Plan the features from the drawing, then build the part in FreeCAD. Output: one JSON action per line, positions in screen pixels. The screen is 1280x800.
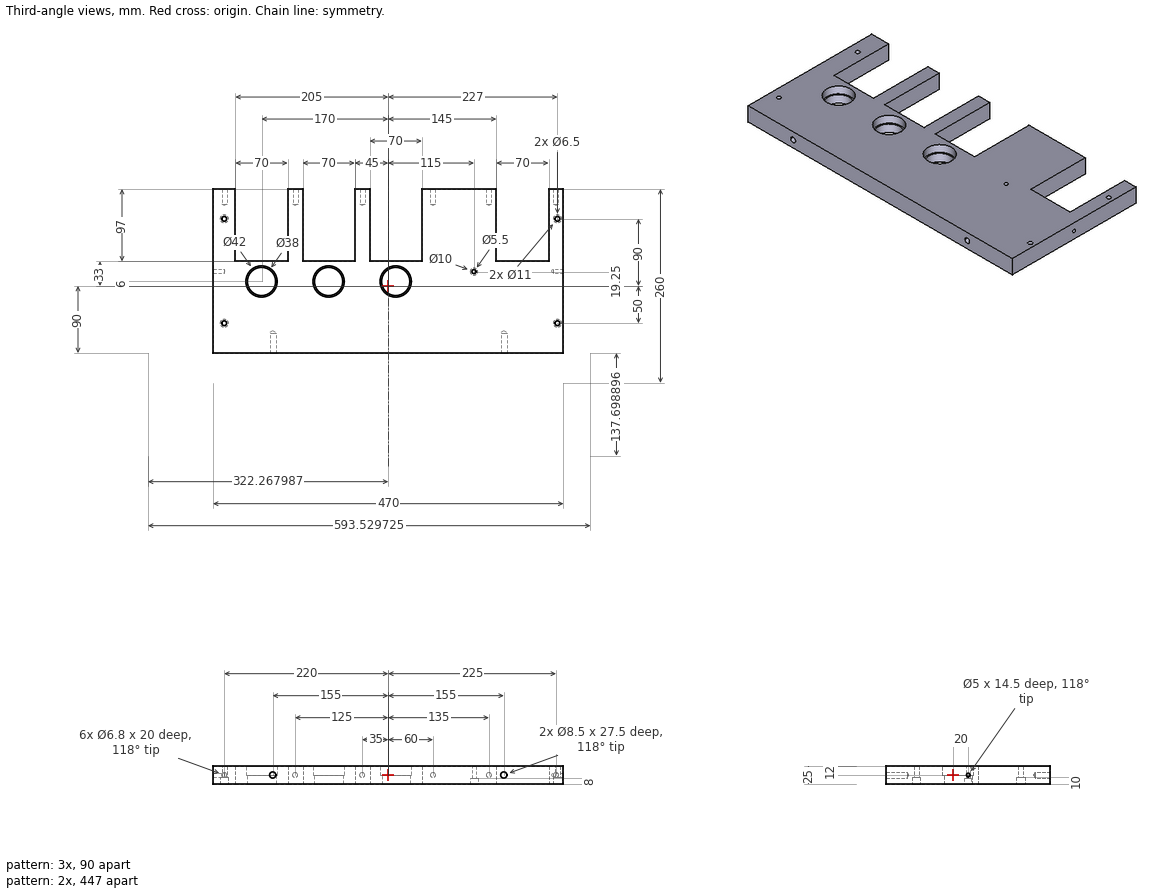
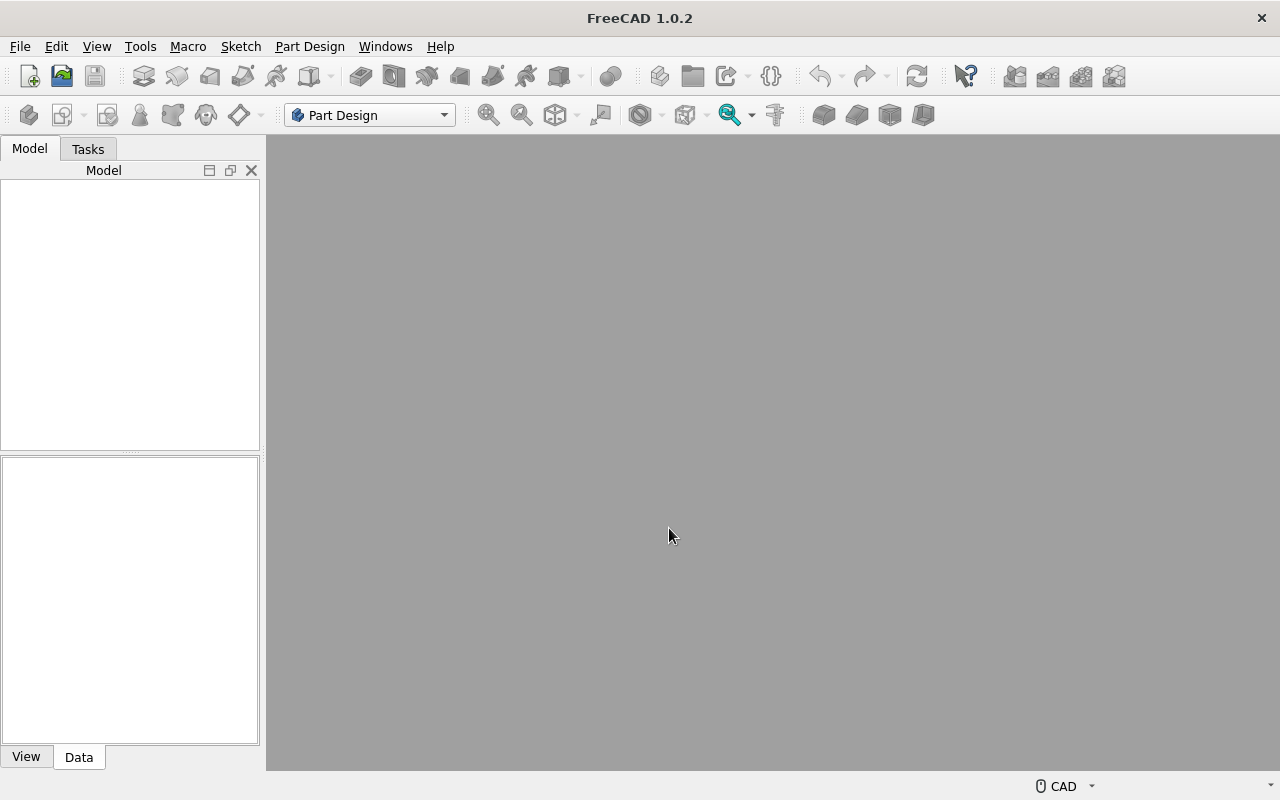
{"action": "left_click", "coordinate": [29, 76]}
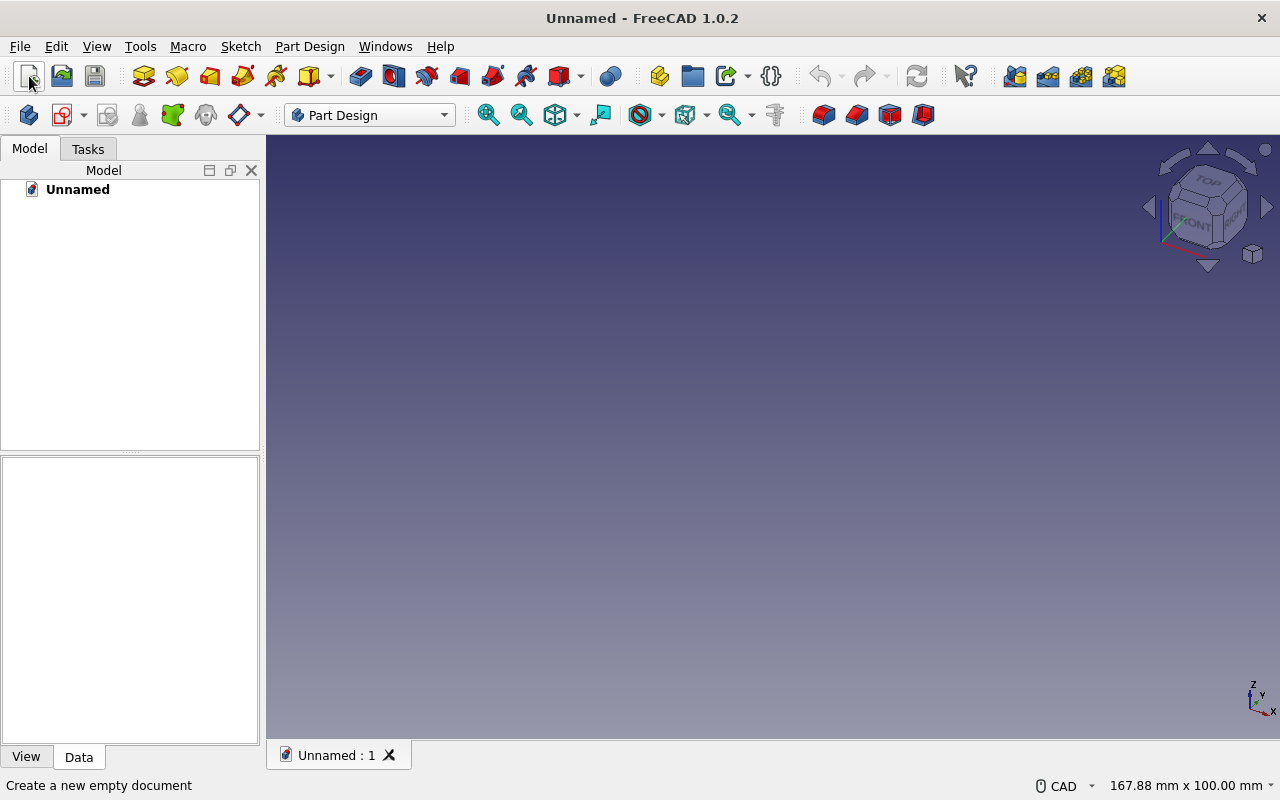
{"action": "left_click", "coordinate": [62, 116]}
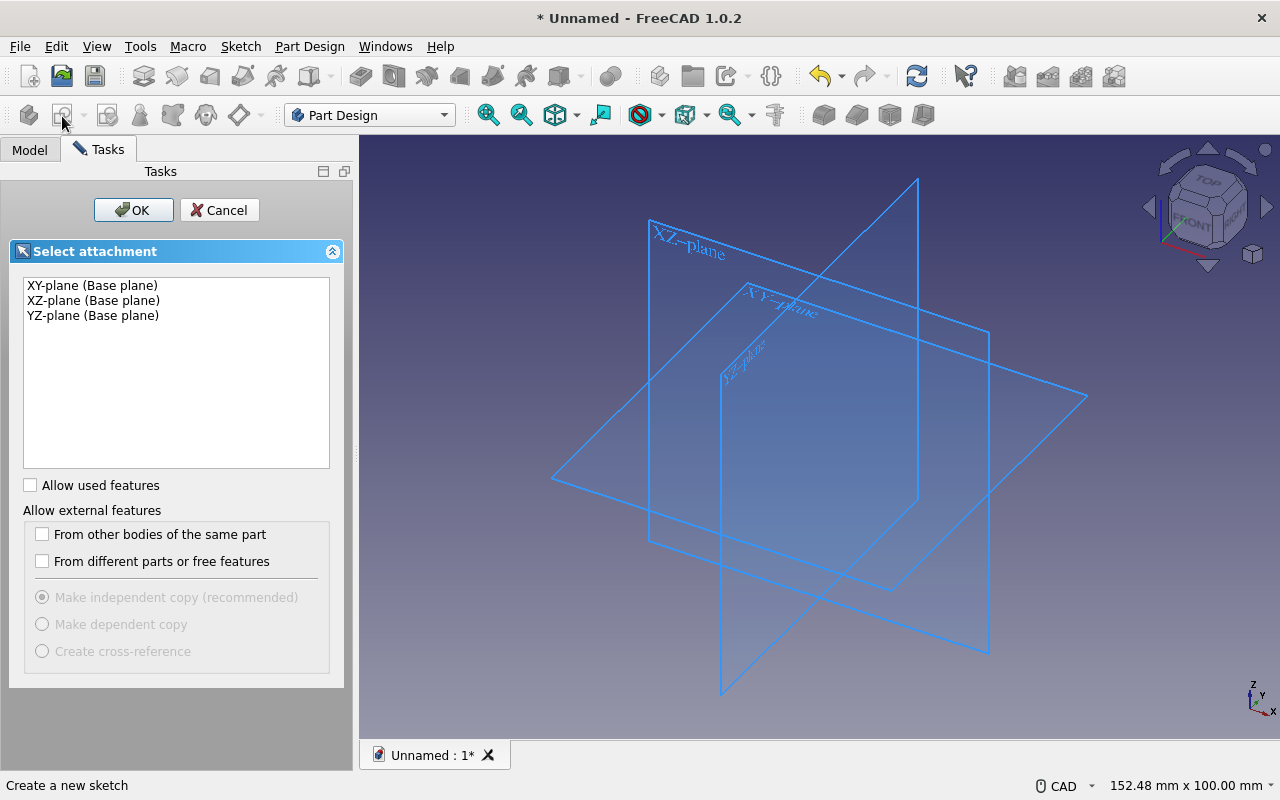
{"action": "left_click", "coordinate": [84, 286]}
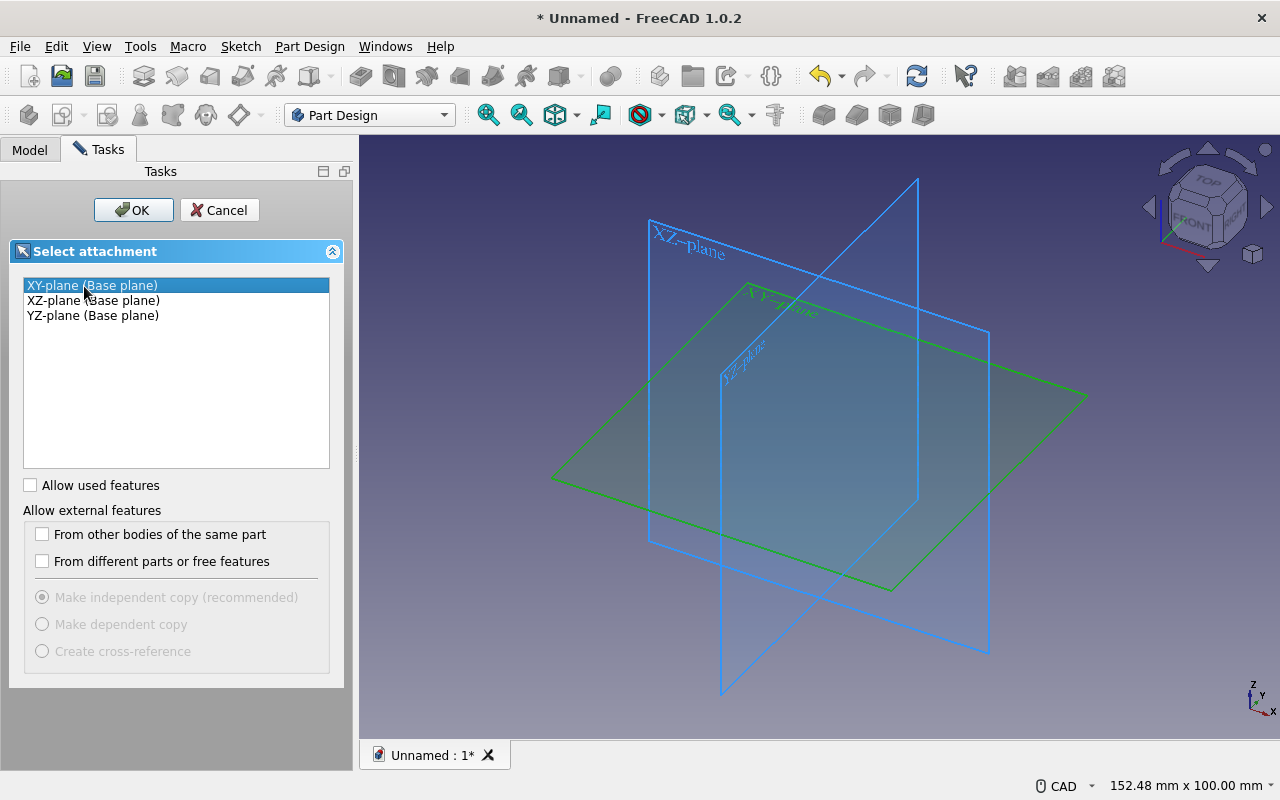
{"action": "left_click", "coordinate": [134, 210]}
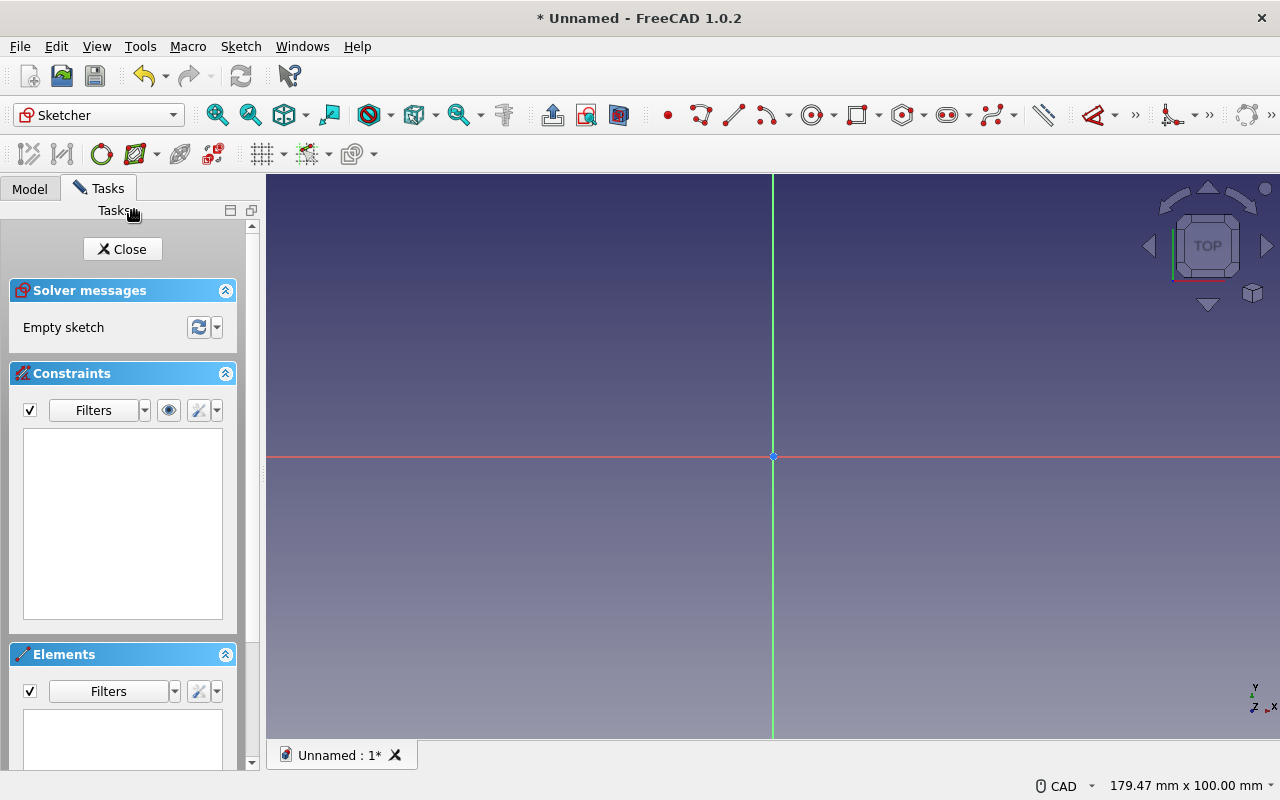
{"action": "scroll", "coordinate": [687, 456], "scroll_direction": "down", "scroll_amount": 8}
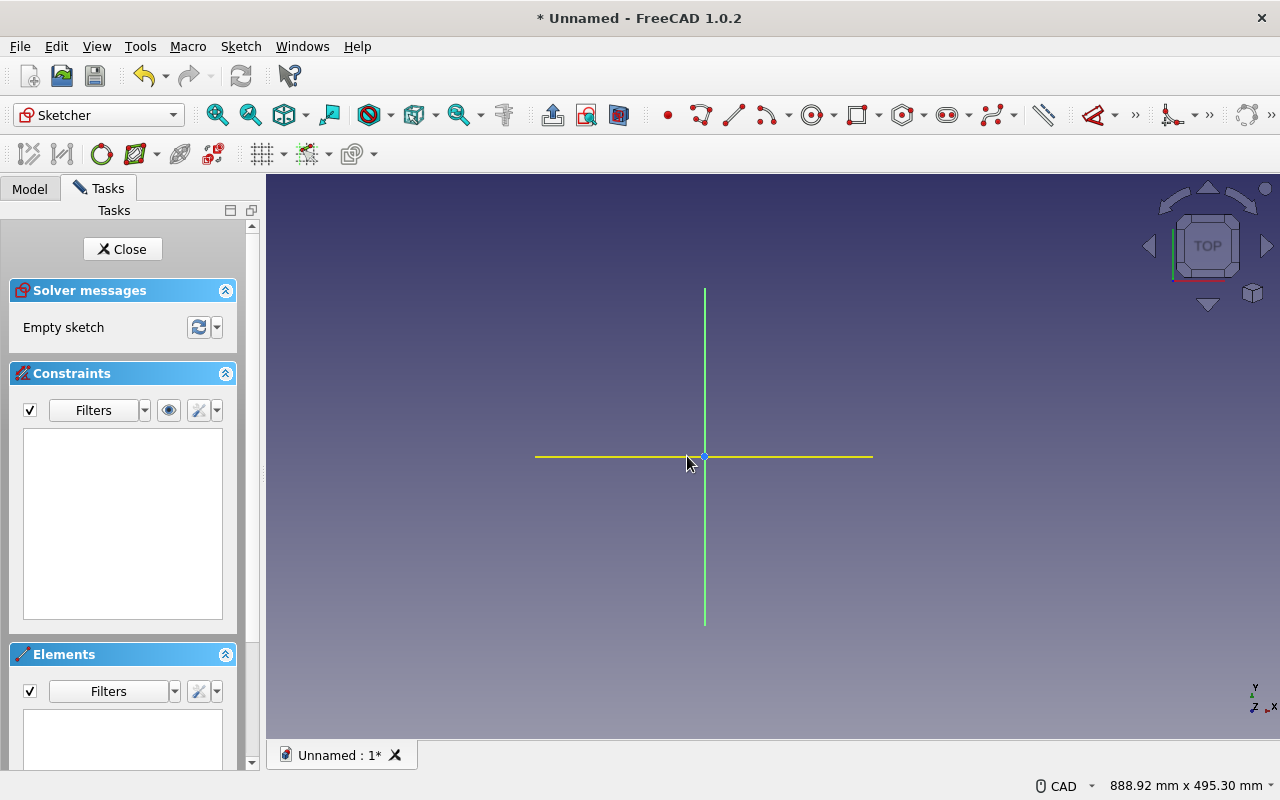
{"action": "left_click", "coordinate": [878, 116]}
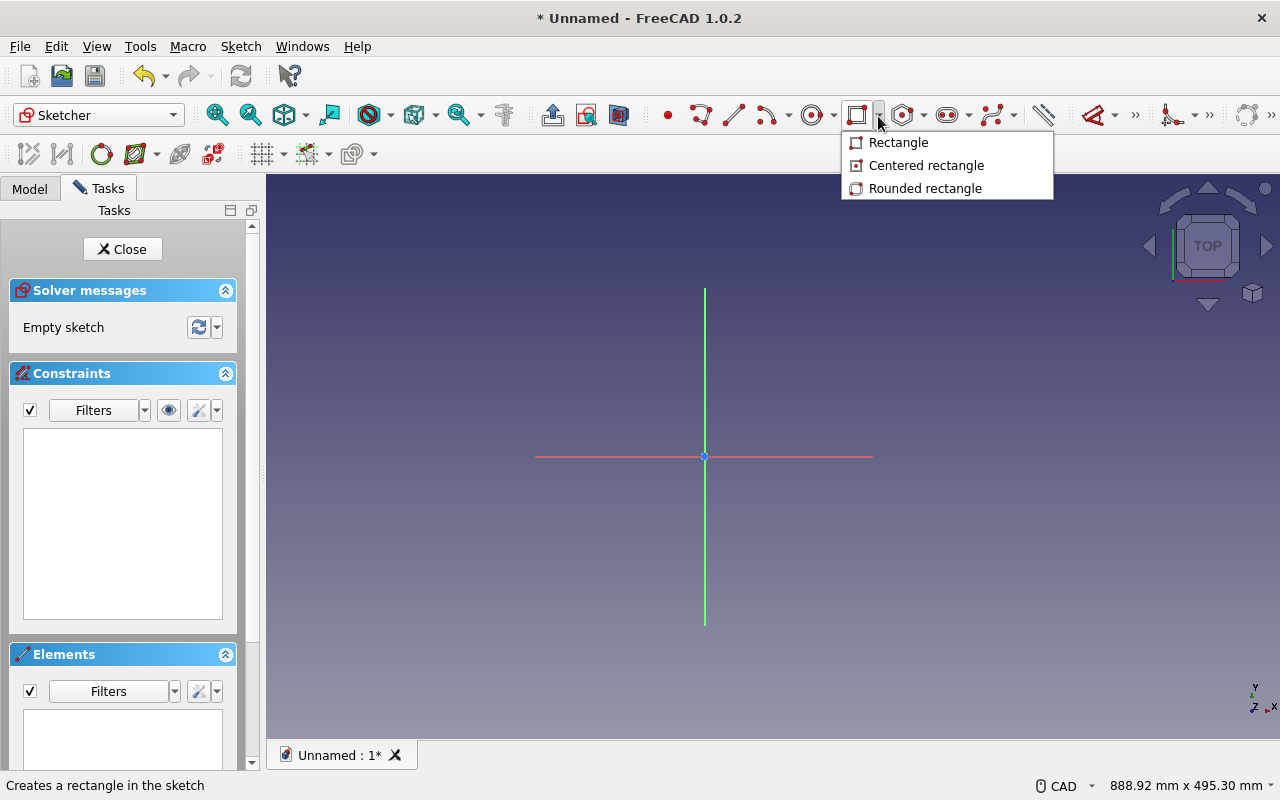
{"action": "left_click", "coordinate": [948, 166]}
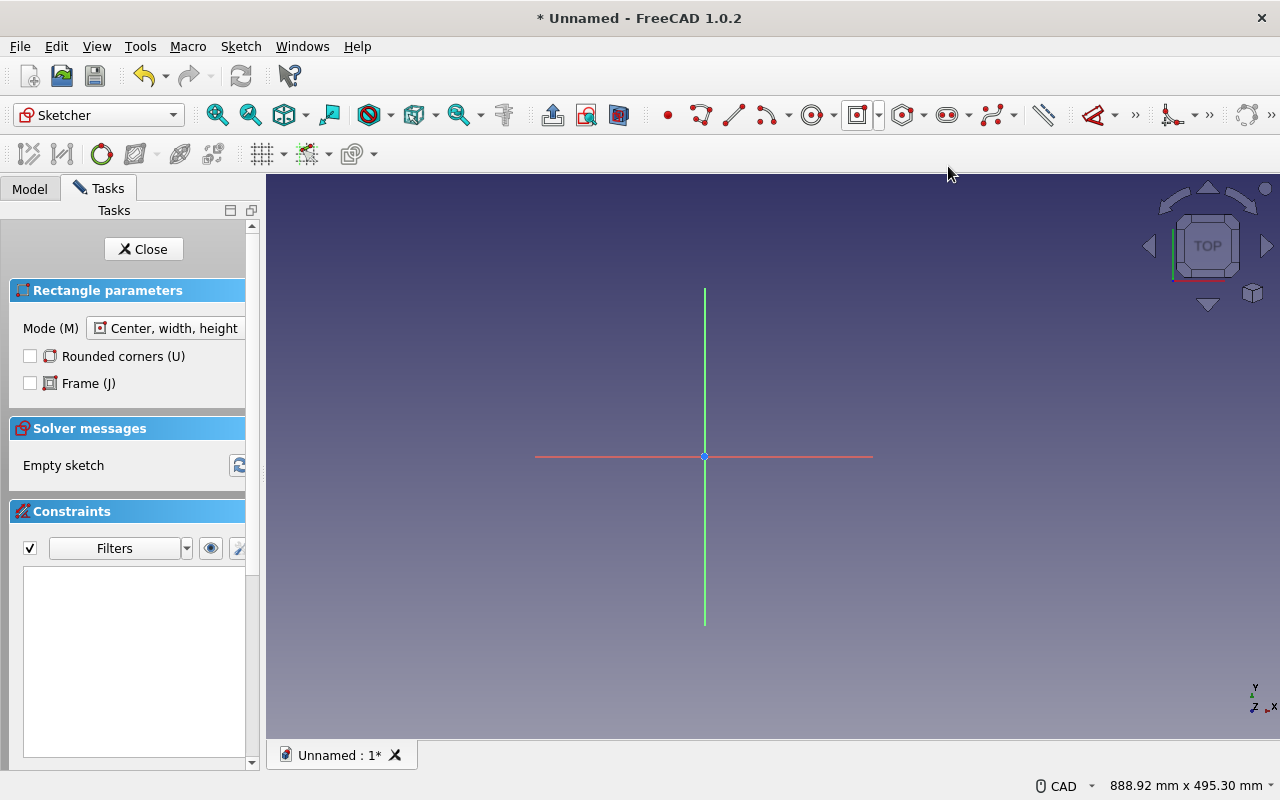
{"action": "left_click", "coordinate": [705, 456]}
{"action": "mouse_move", "coordinate": [973, 308]}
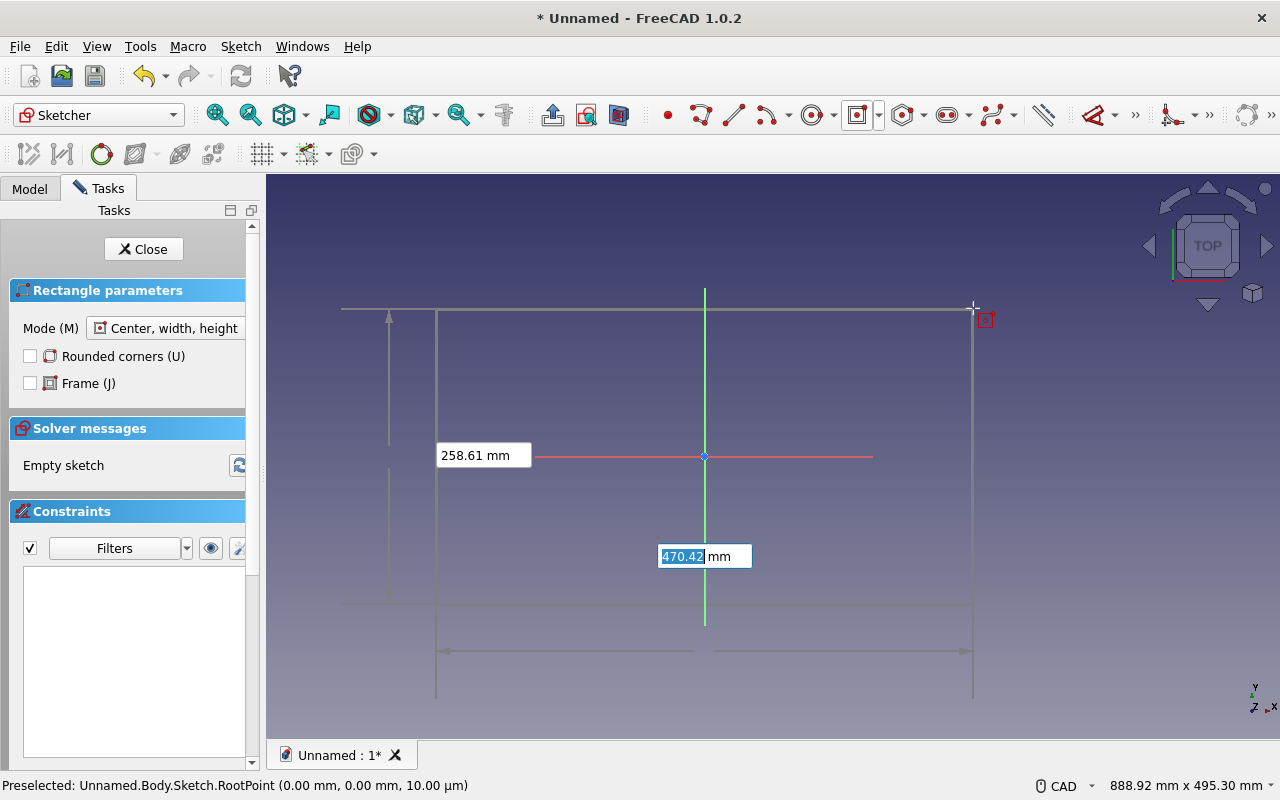
{"action": "type", "text": "470"}
{"action": "key", "text": "Tab"}
{"action": "type", "text": "260"}
{"action": "key", "text": "Return"}
{"action": "key", "text": "Escape"}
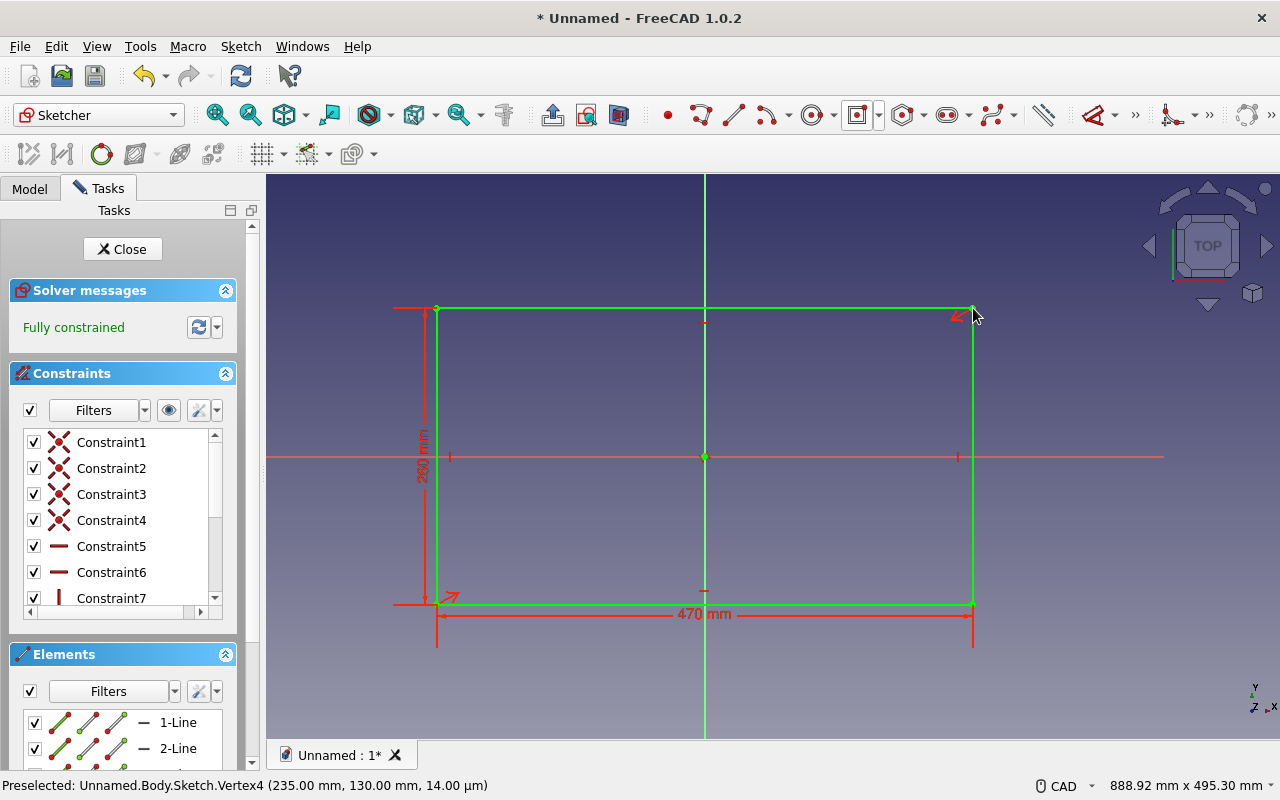
{"action": "left_click", "coordinate": [123, 249]}